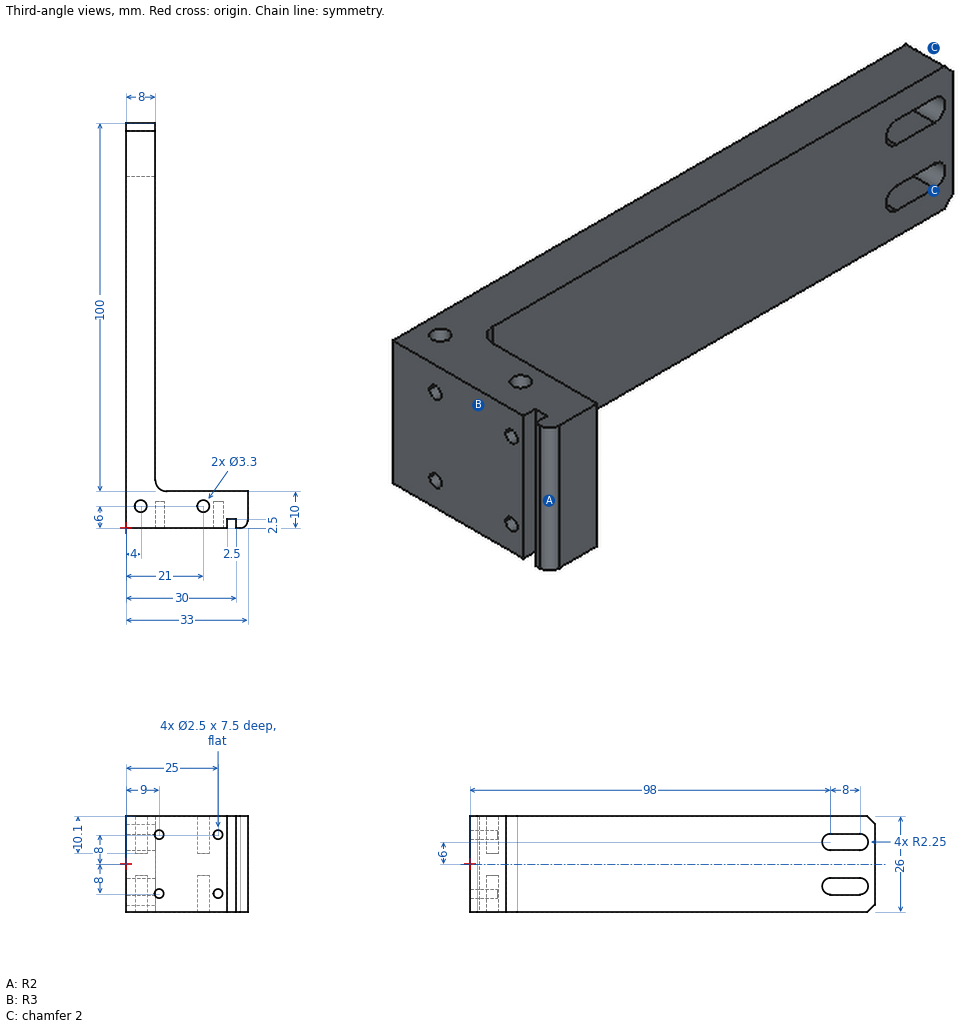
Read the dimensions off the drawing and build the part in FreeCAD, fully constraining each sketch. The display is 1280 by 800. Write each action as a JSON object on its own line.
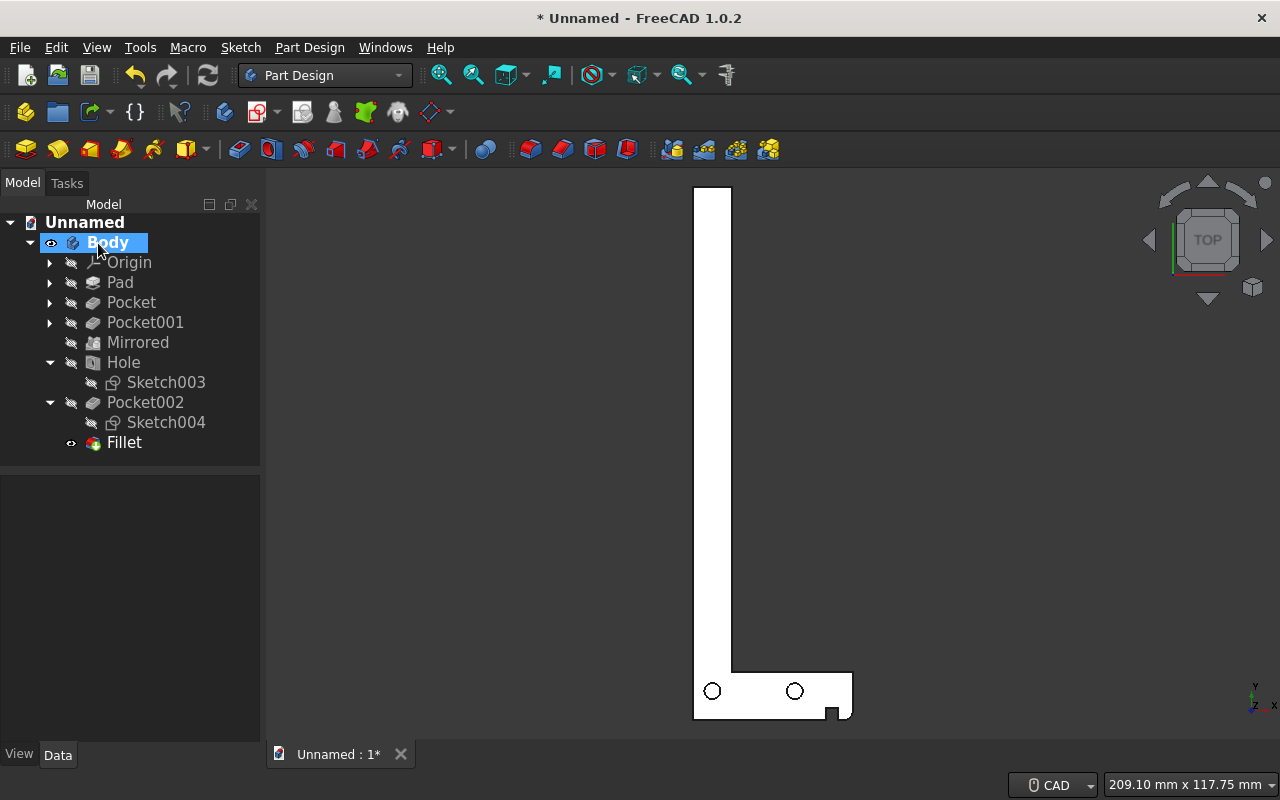
{"action": "key", "text": "1"}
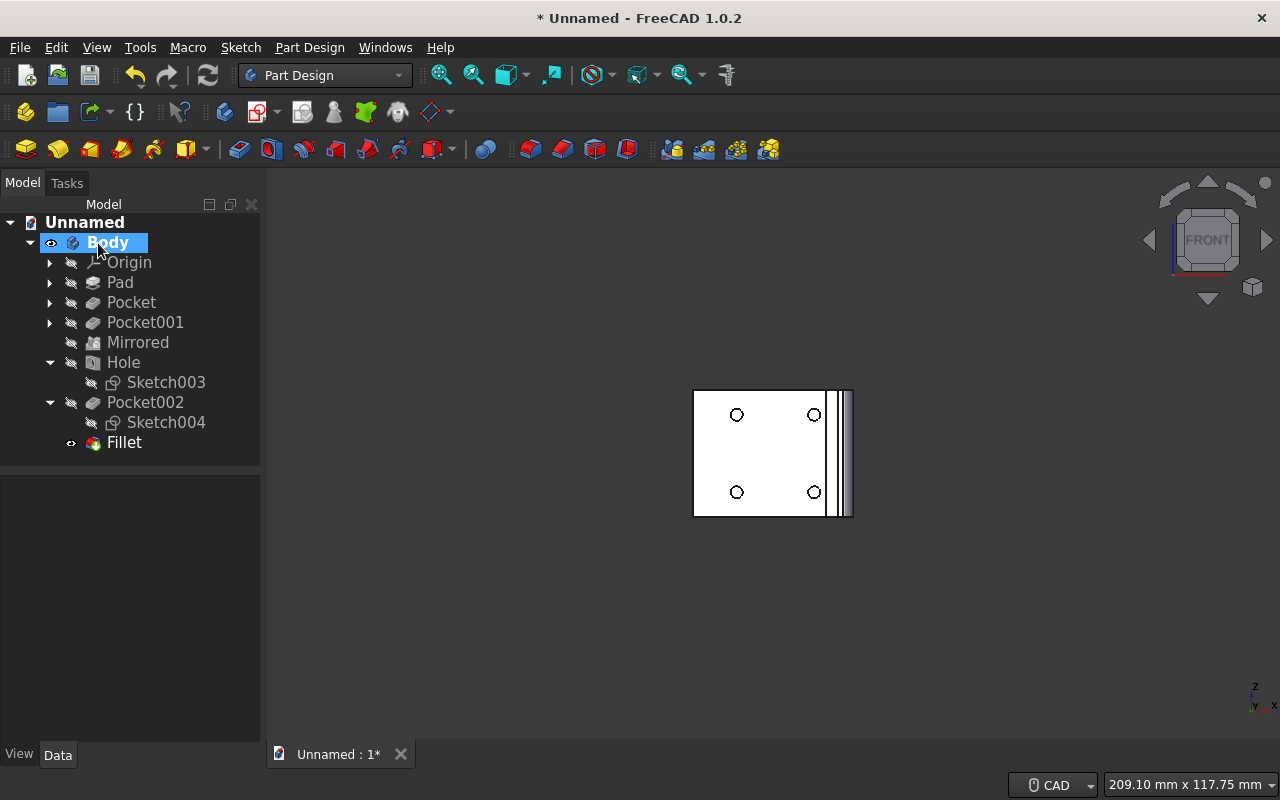
{"action": "left_click", "coordinate": [442, 76]}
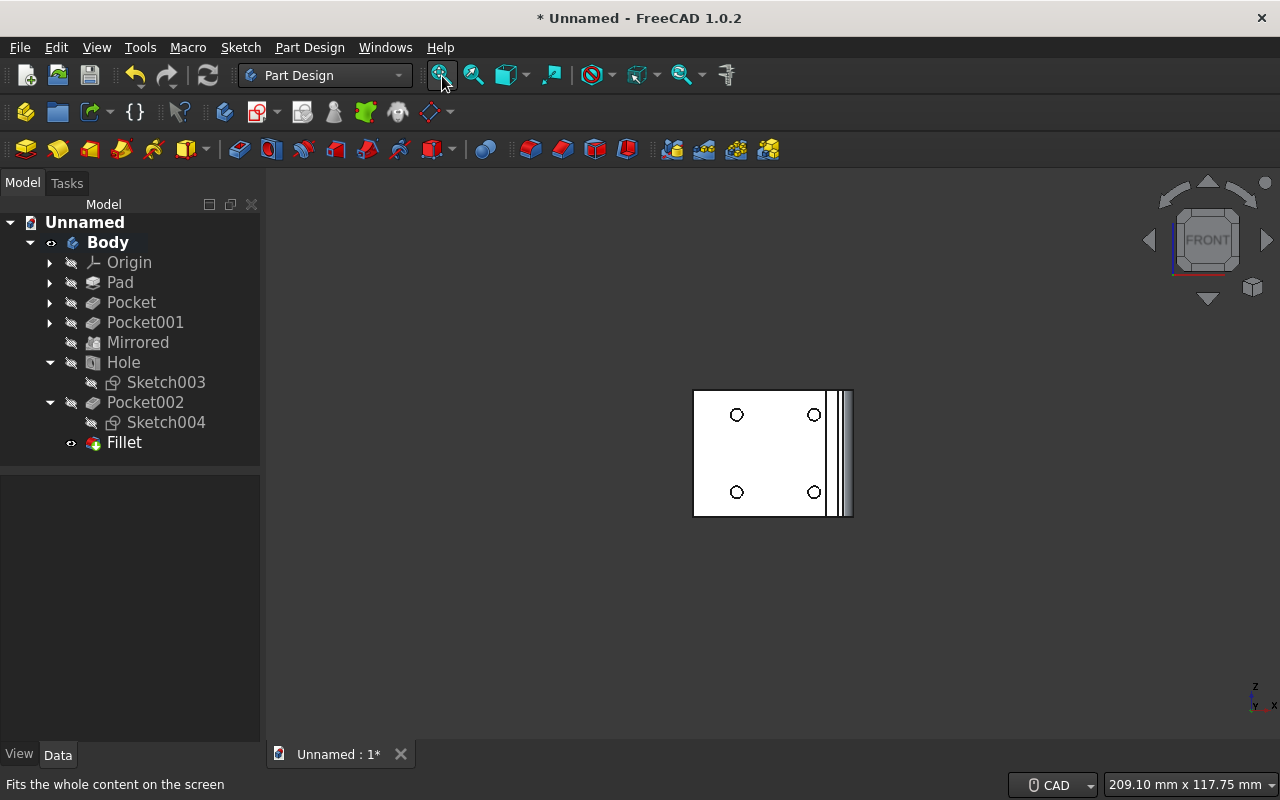
{"action": "key", "text": "3"}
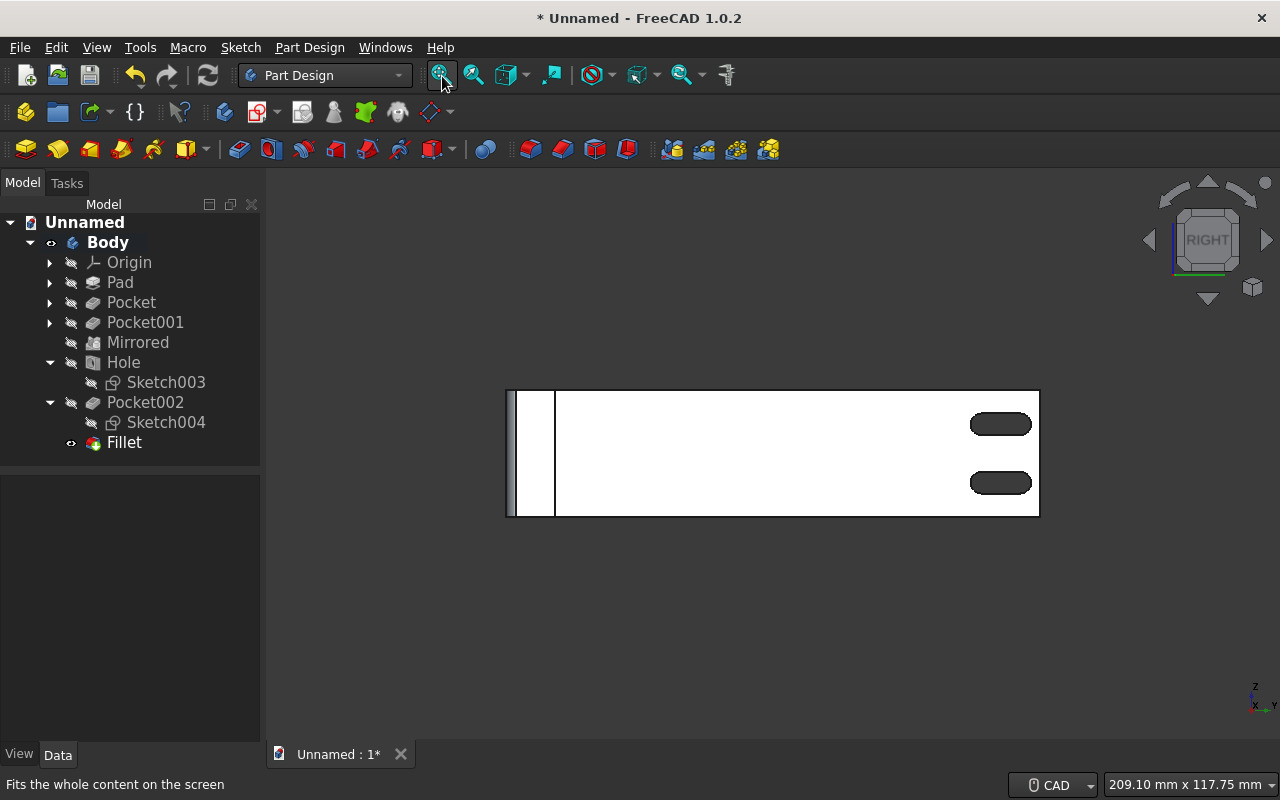
{"action": "key", "text": "5"}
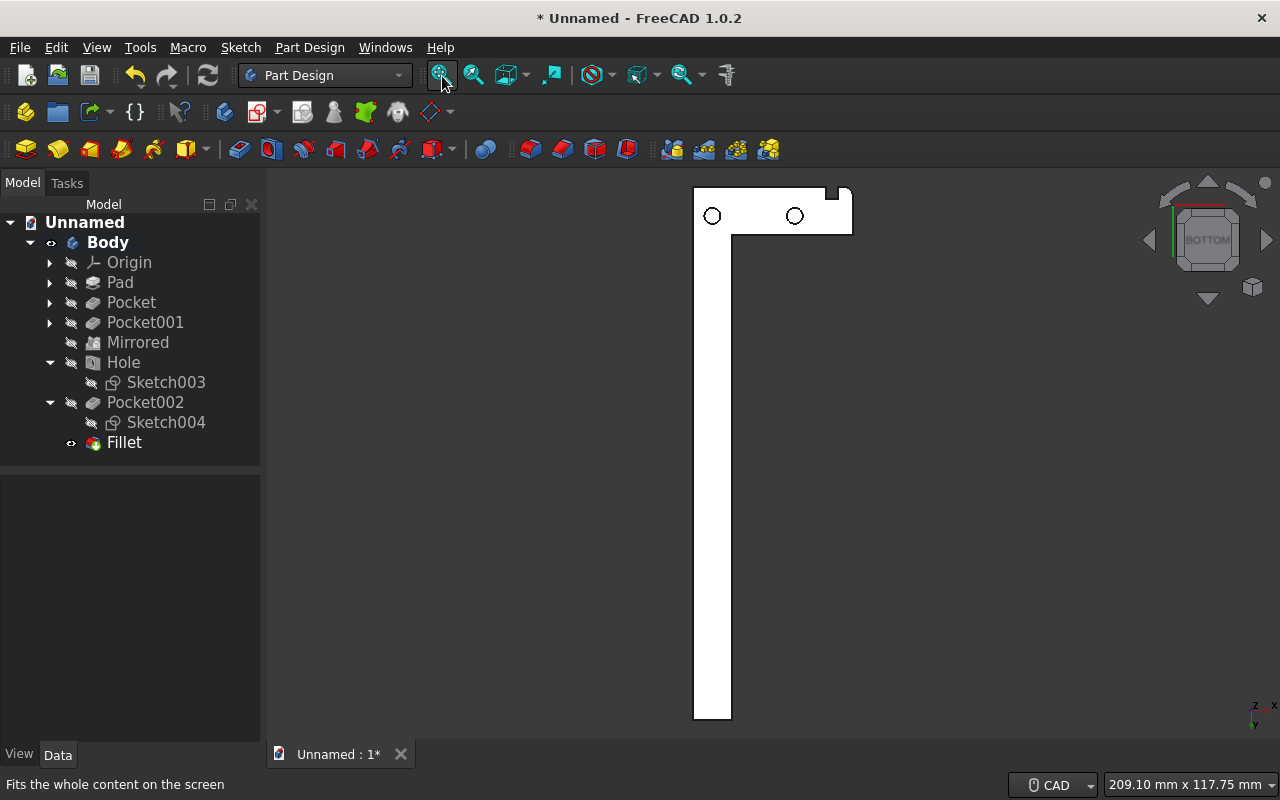
{"action": "key", "text": "4"}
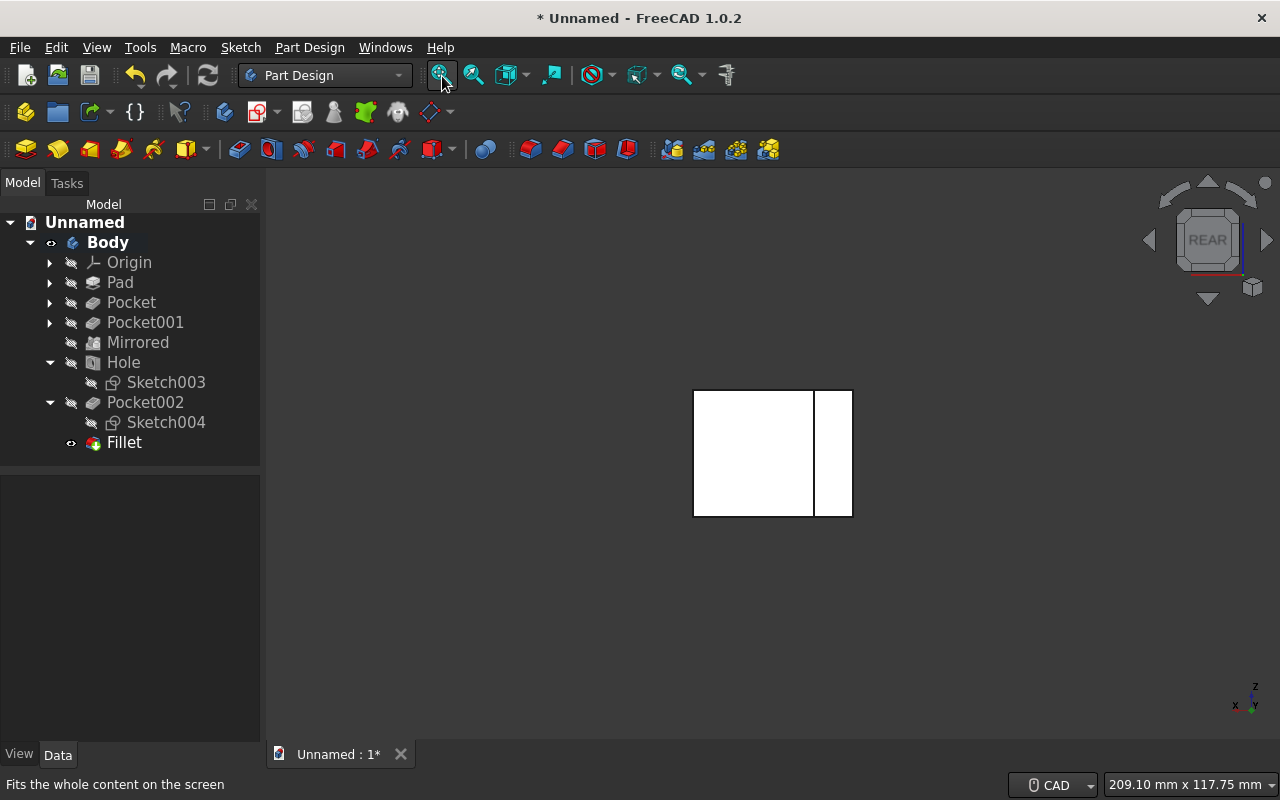
{"action": "left_click", "coordinate": [442, 76]}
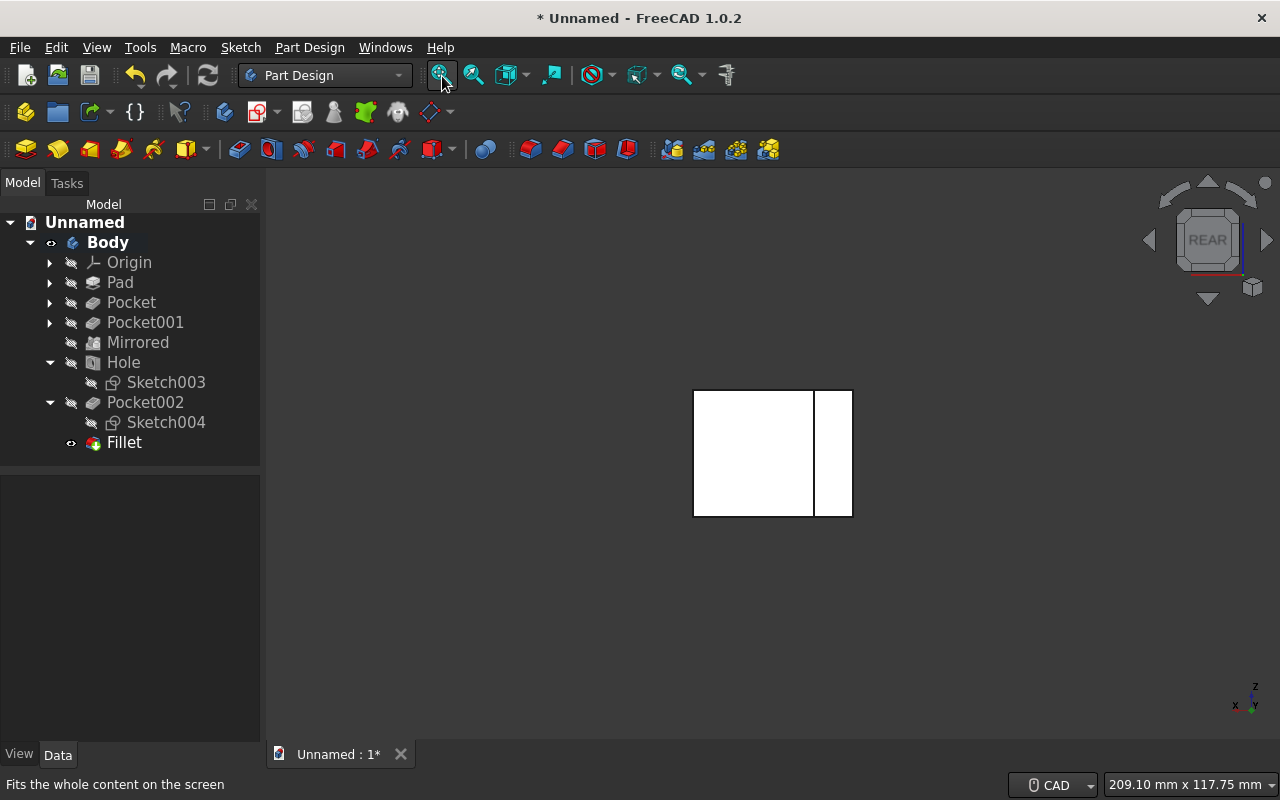
{"action": "key", "text": "6"}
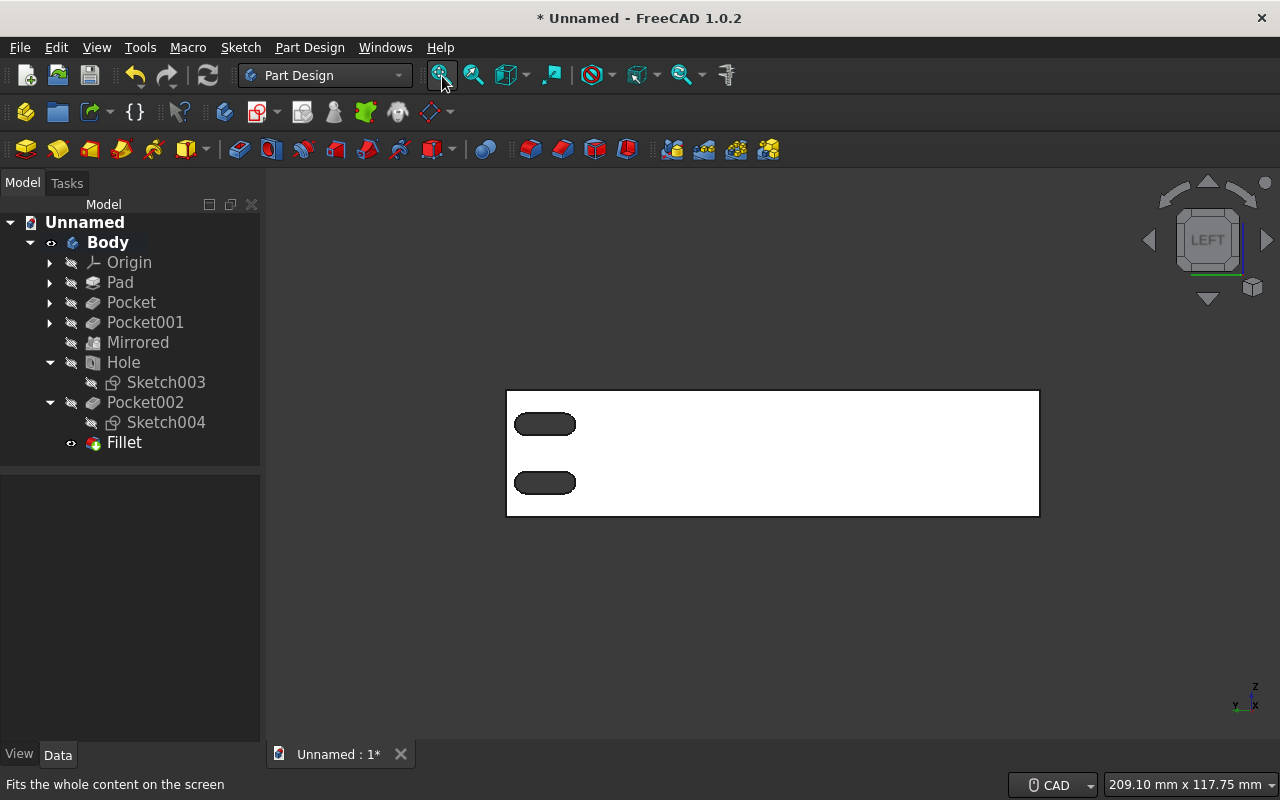
{"action": "key", "text": "v 3"}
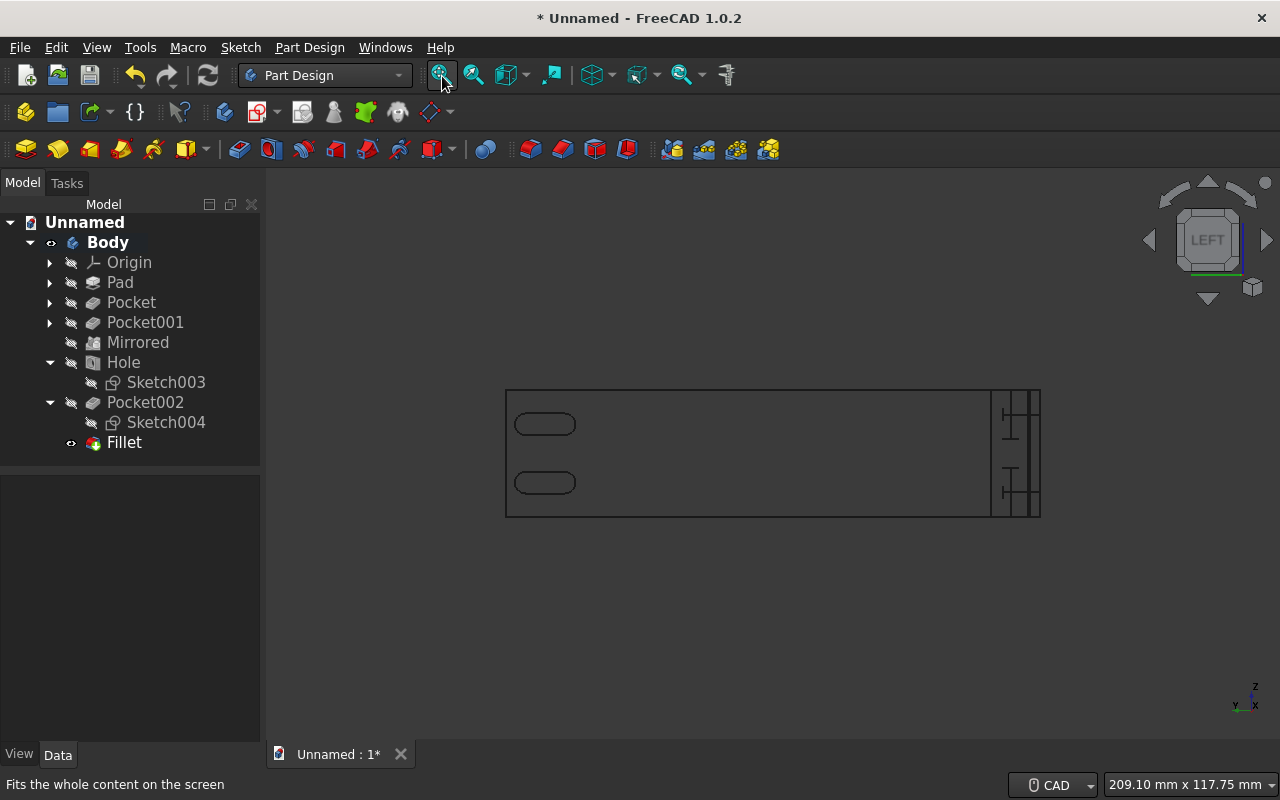
{"action": "key", "text": "0"}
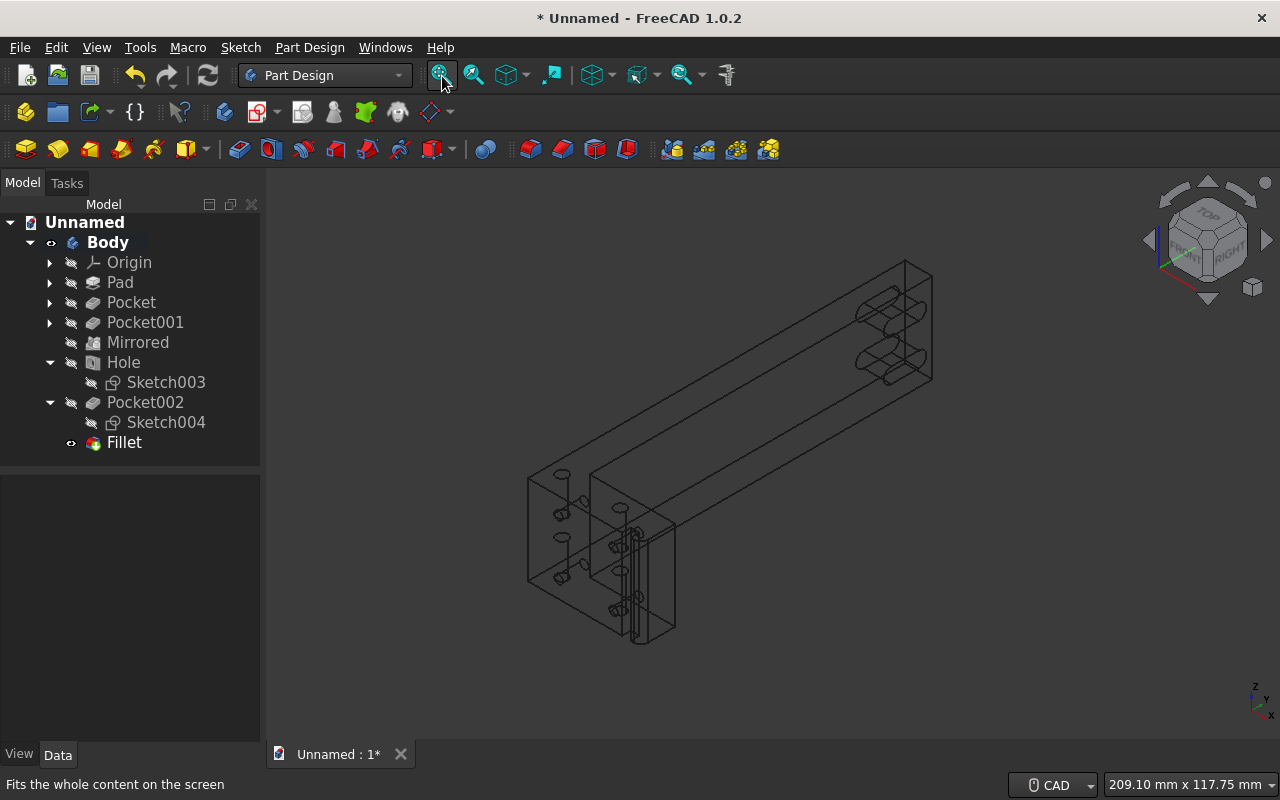
{"action": "left_click", "coordinate": [590, 525]}